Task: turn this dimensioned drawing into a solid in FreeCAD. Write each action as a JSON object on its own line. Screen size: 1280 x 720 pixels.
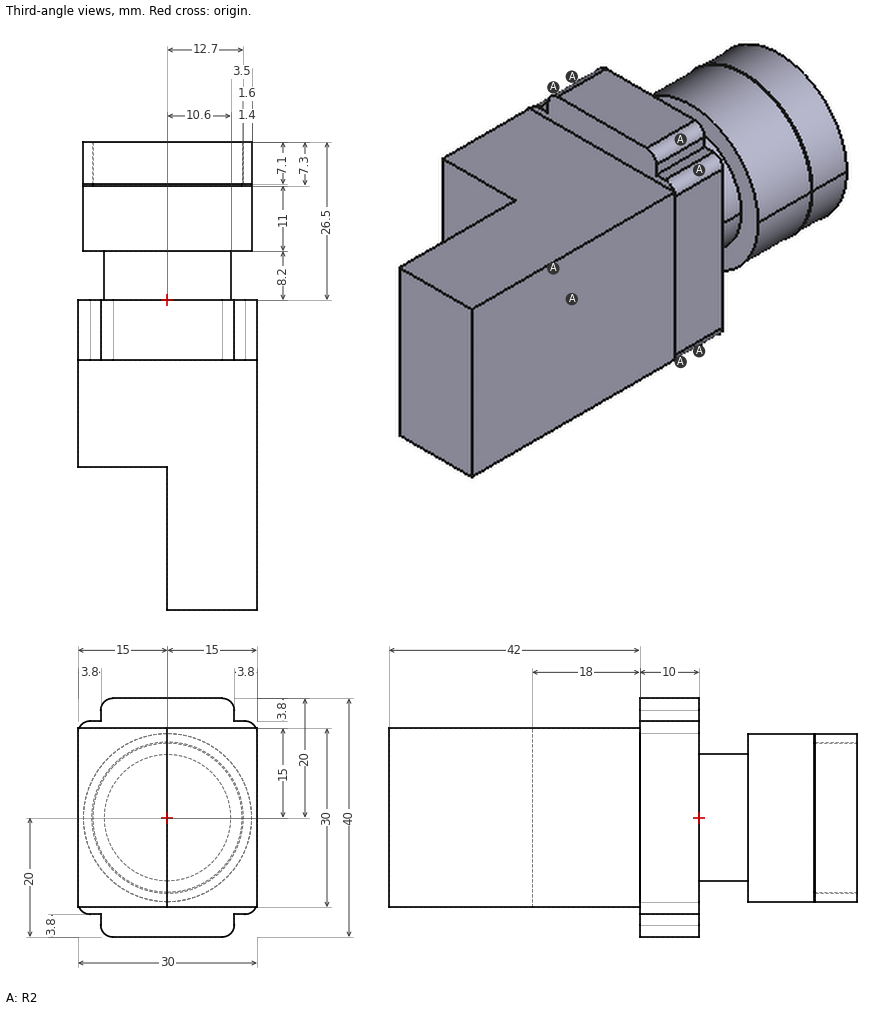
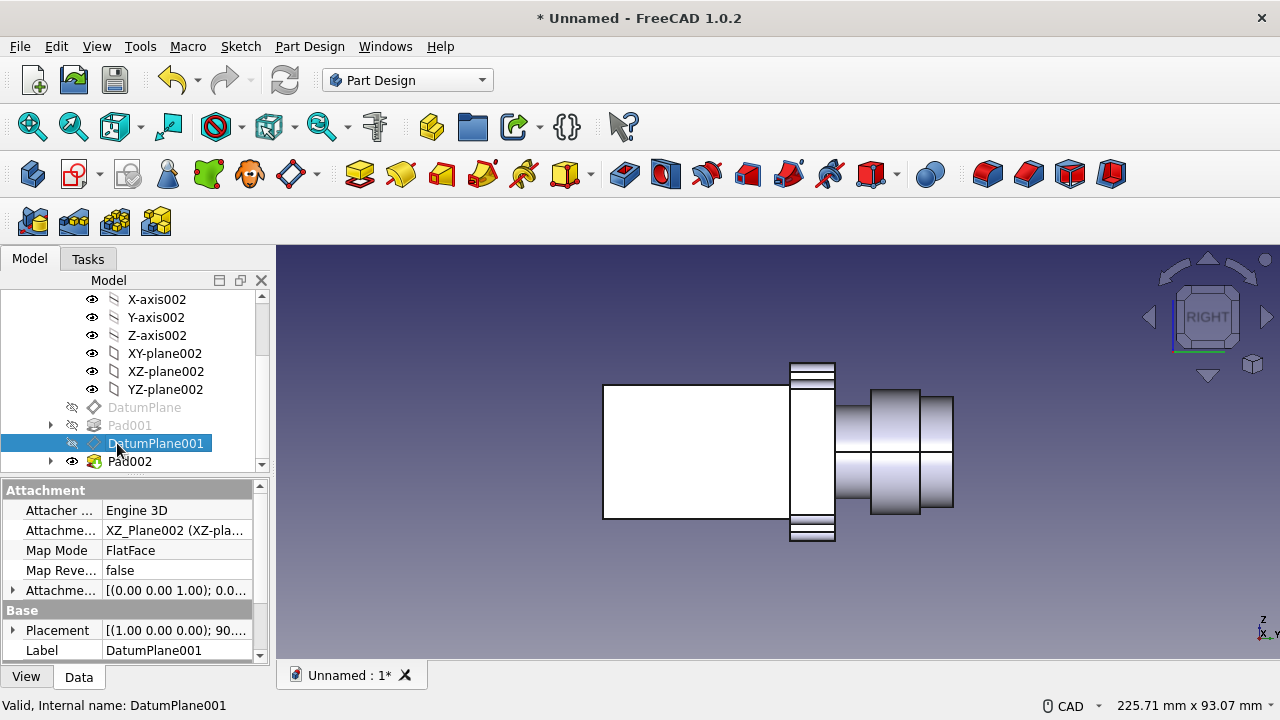
{"action": "left_click", "coordinate": [33, 128]}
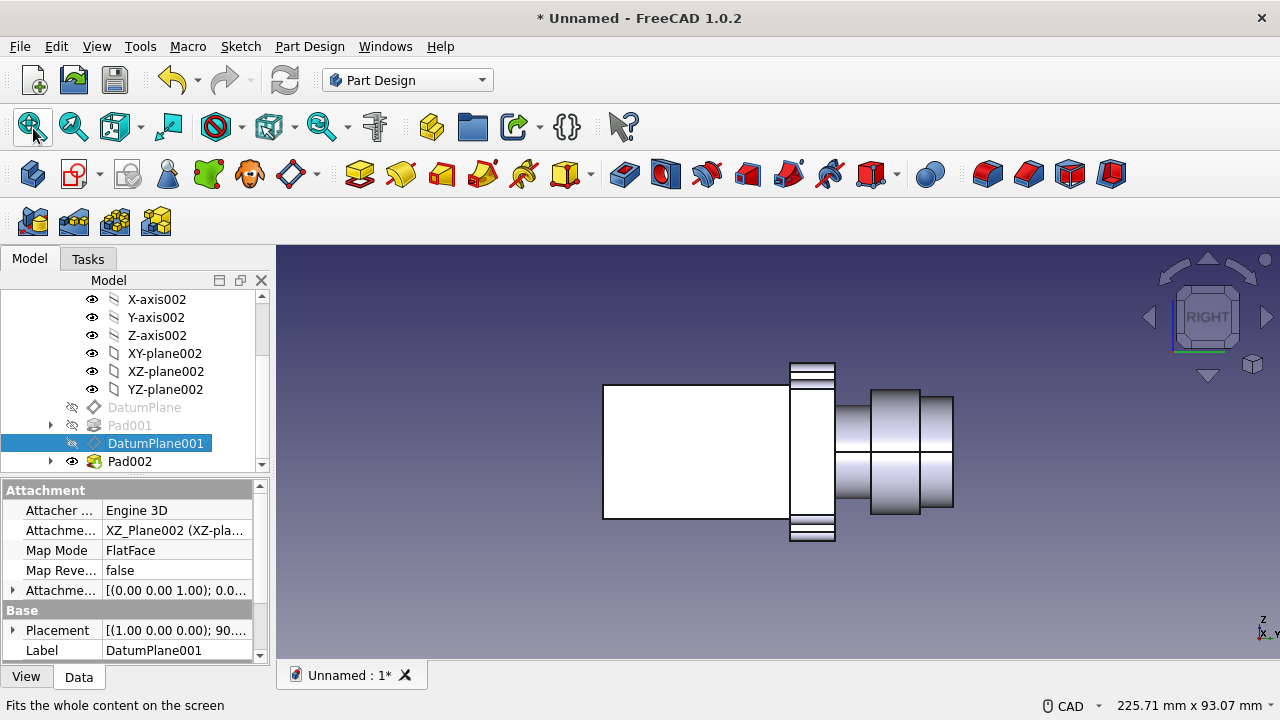
{"action": "left_click", "coordinate": [316, 619]}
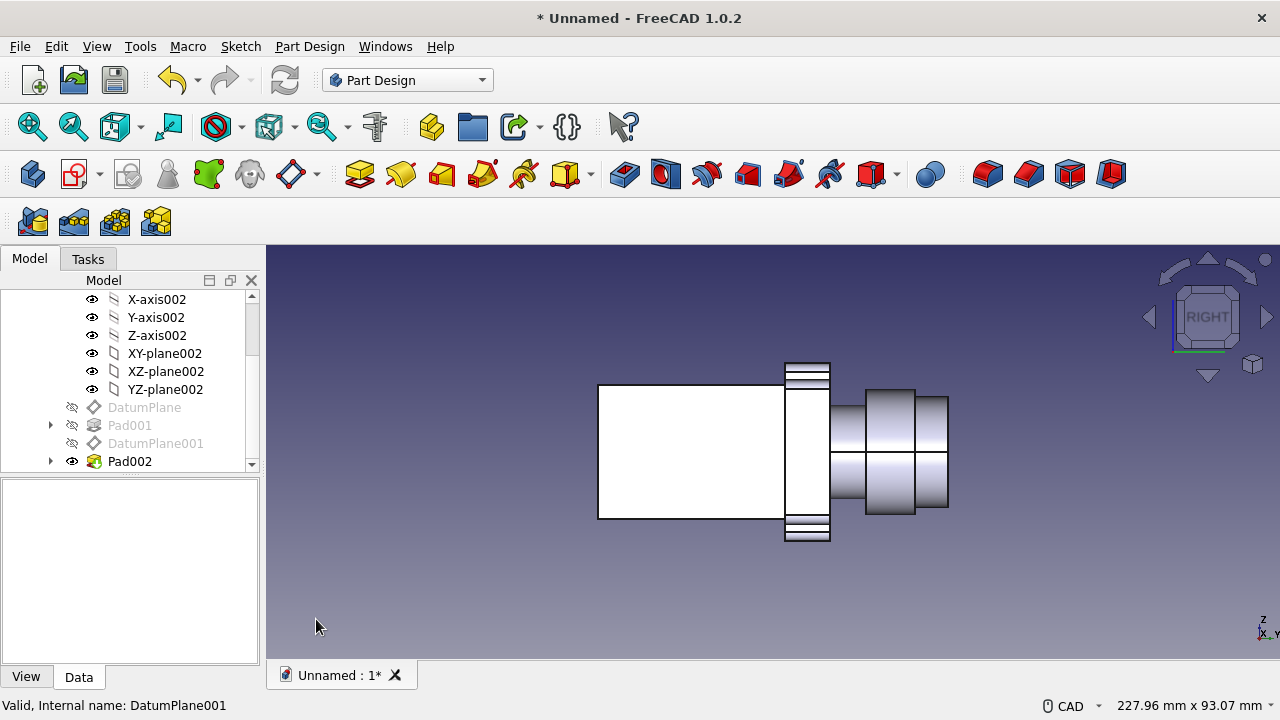
{"action": "left_click", "coordinate": [33, 174]}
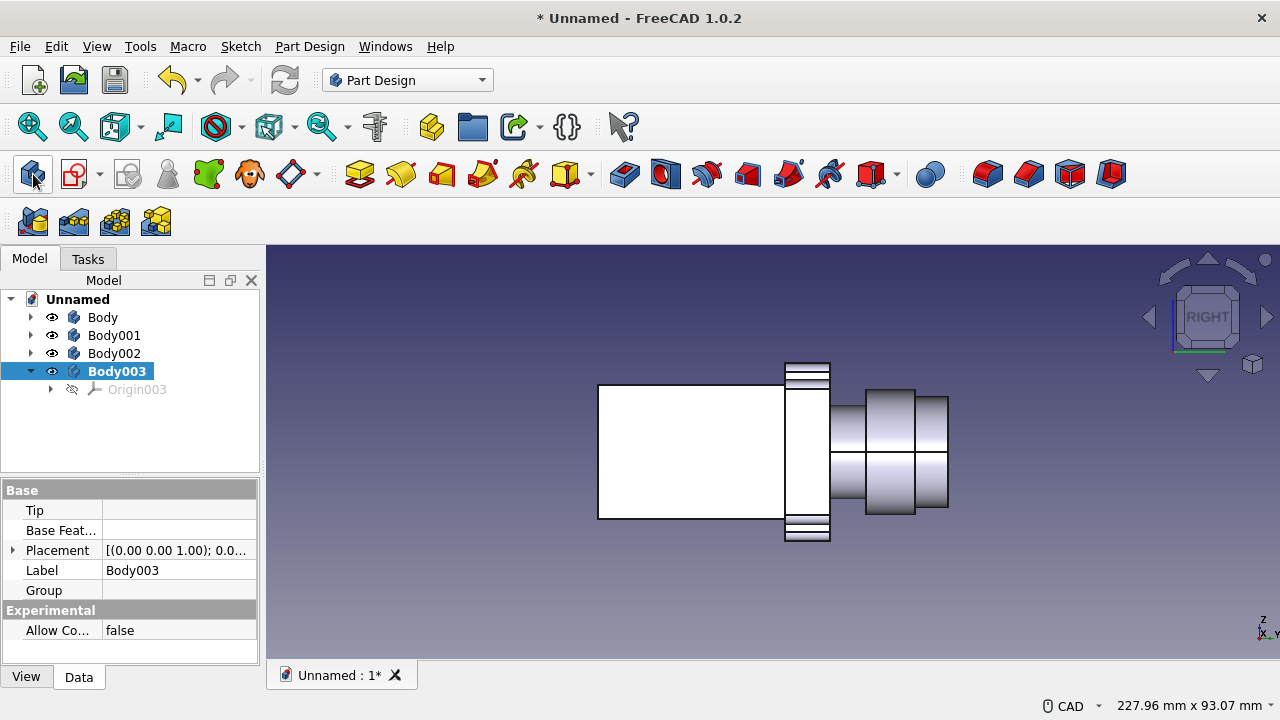
{"action": "left_click", "coordinate": [306, 619]}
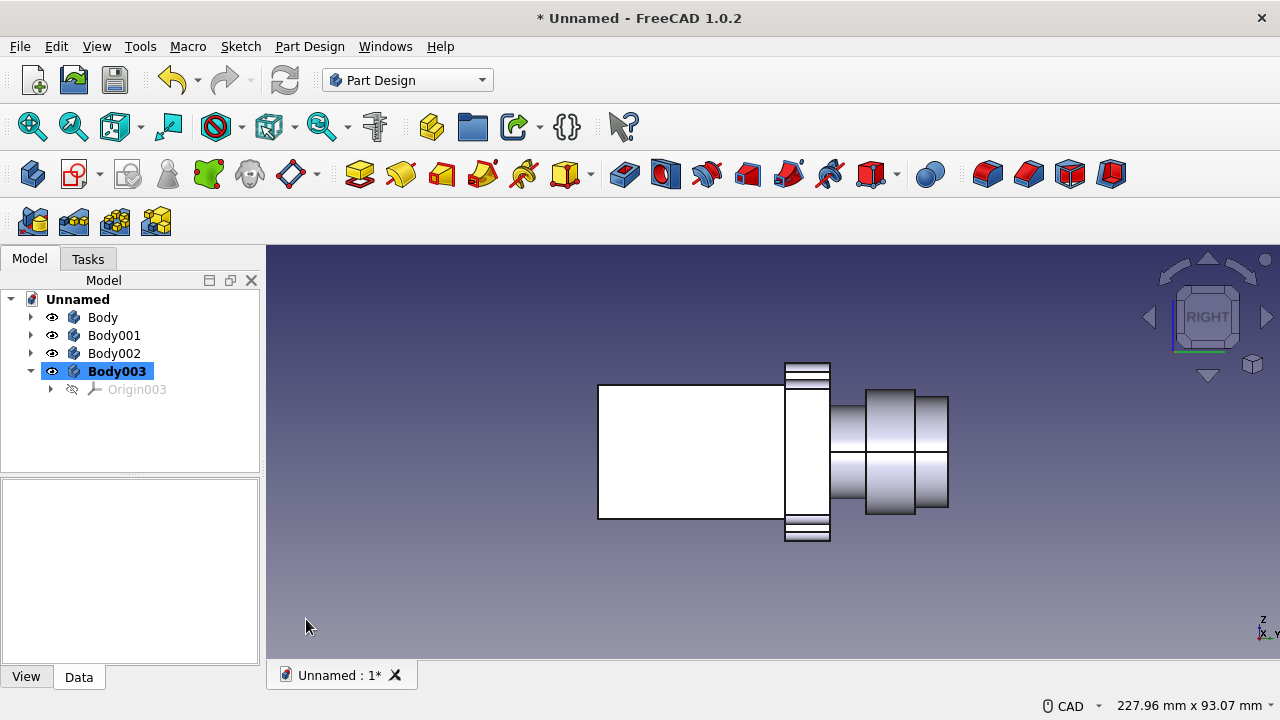
{"action": "left_click", "coordinate": [74, 174]}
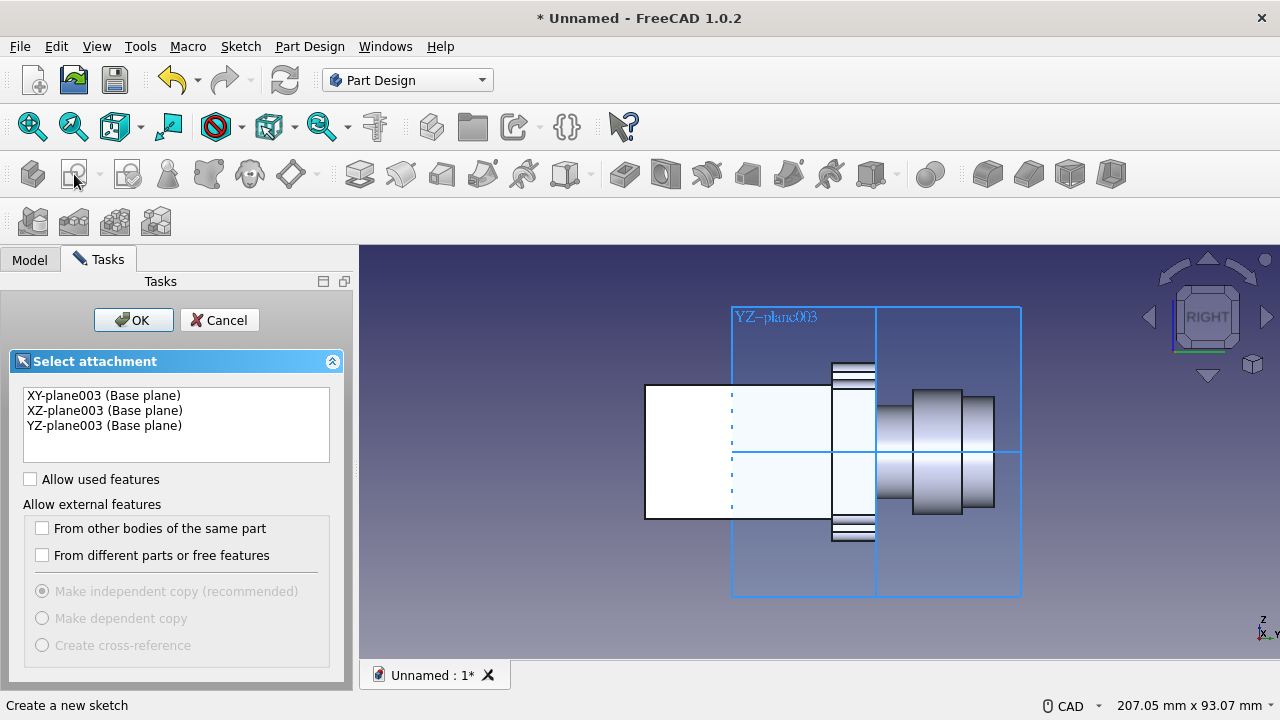
{"action": "left_click", "coordinate": [84, 396]}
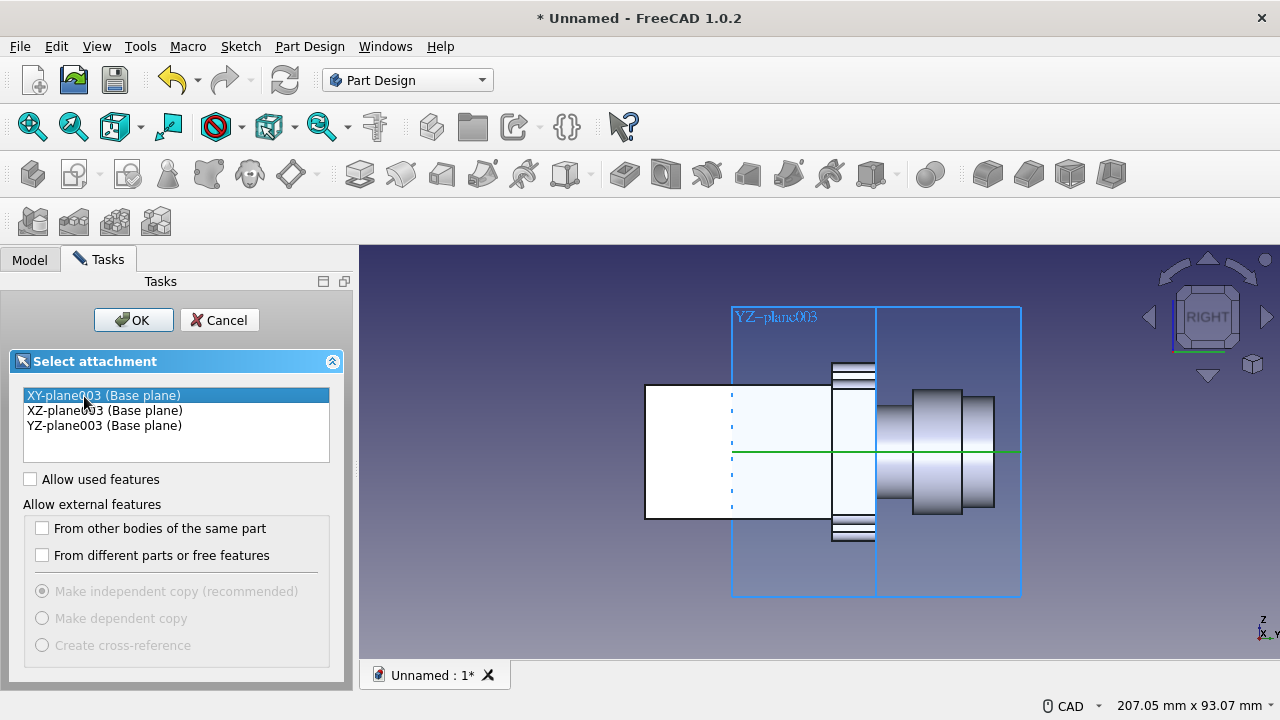
{"action": "left_click", "coordinate": [134, 320]}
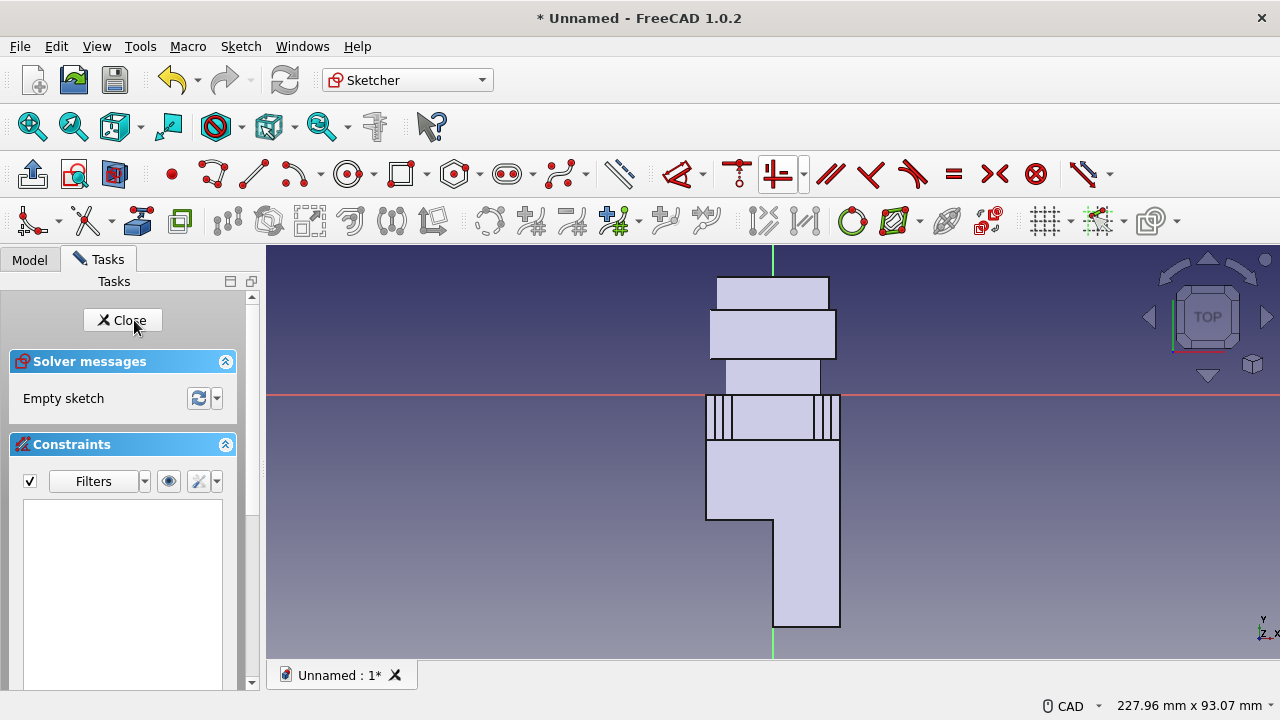
{"action": "scroll", "coordinate": [853, 273], "scroll_direction": "up", "scroll_amount": 10}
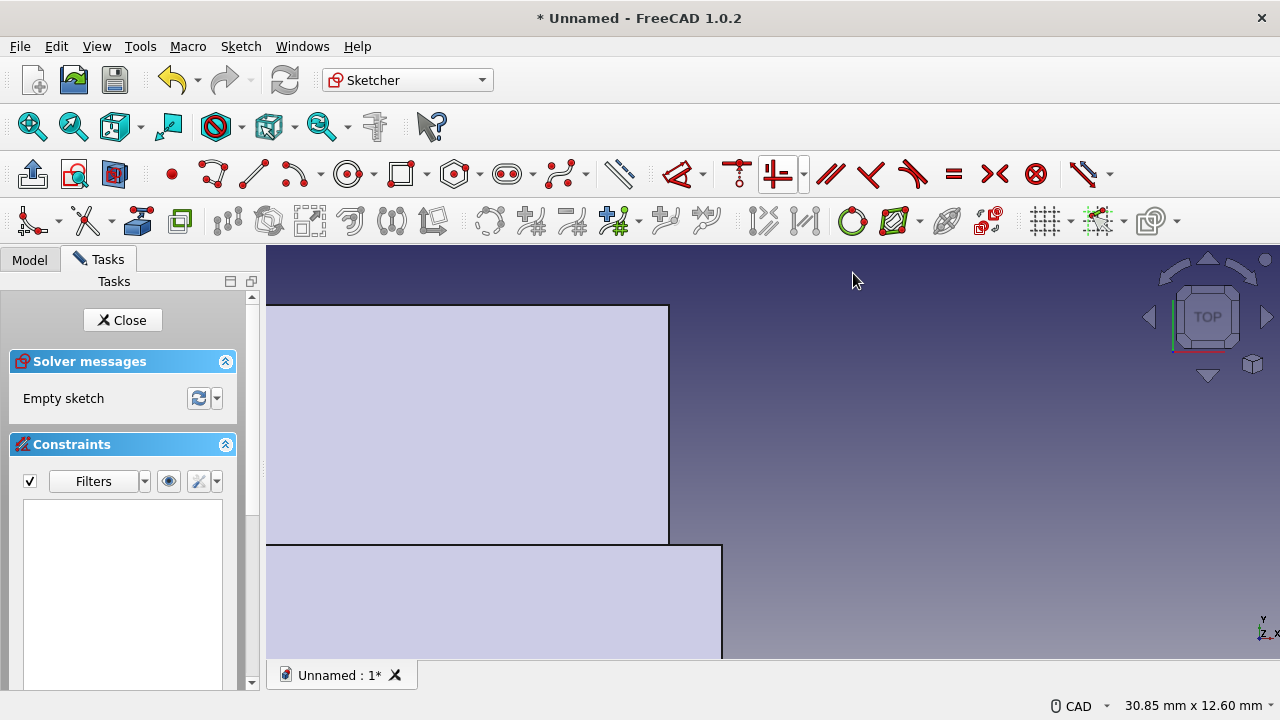
{"action": "left_click", "coordinate": [400, 174]}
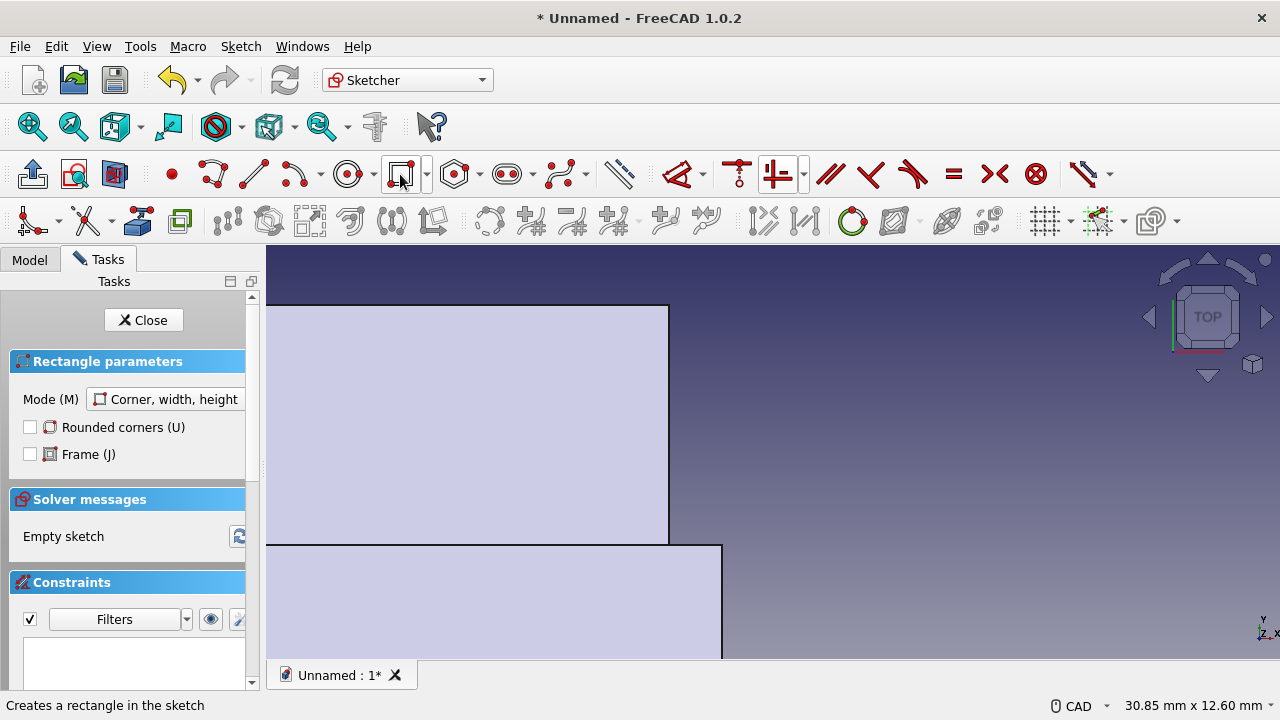
{"action": "left_click", "coordinate": [676, 305]}
{"action": "mouse_move", "coordinate": [722, 539]}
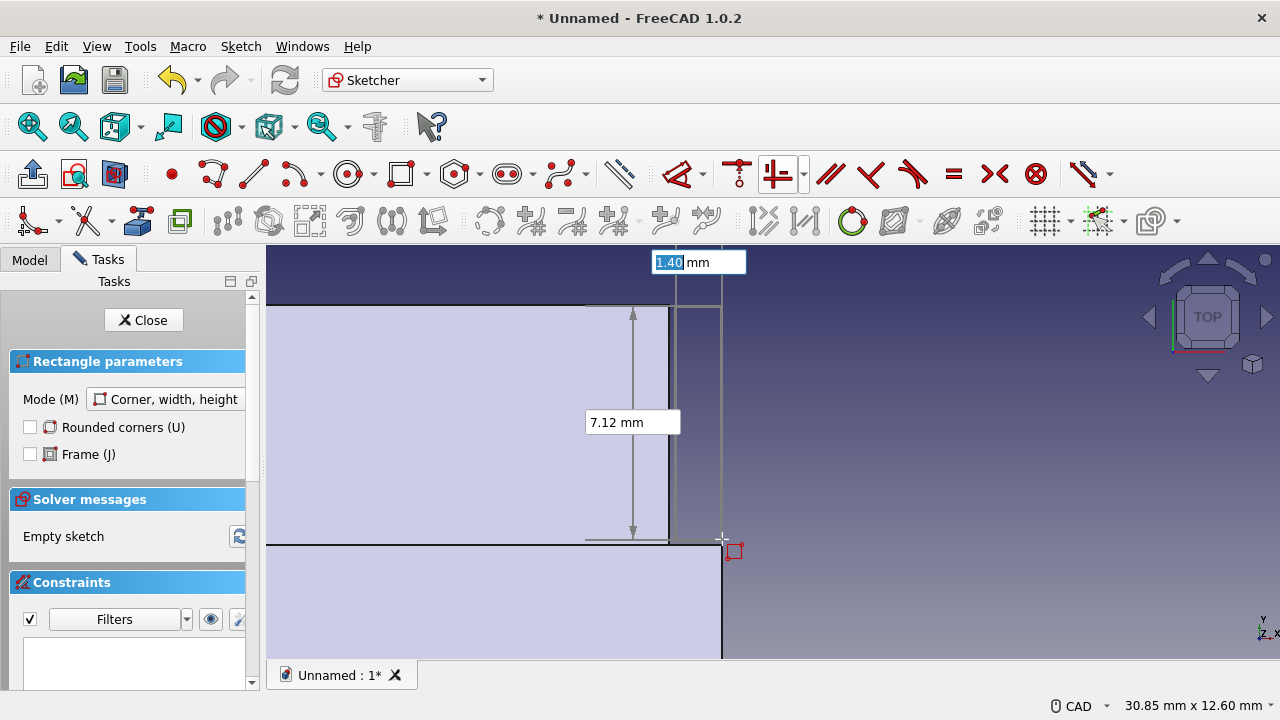
{"action": "type", "text": "1.4"}
{"action": "key", "text": "Tab"}
{"action": "type", "text": "7.1"}
{"action": "key", "text": "Return"}
{"action": "key", "text": "Escape"}